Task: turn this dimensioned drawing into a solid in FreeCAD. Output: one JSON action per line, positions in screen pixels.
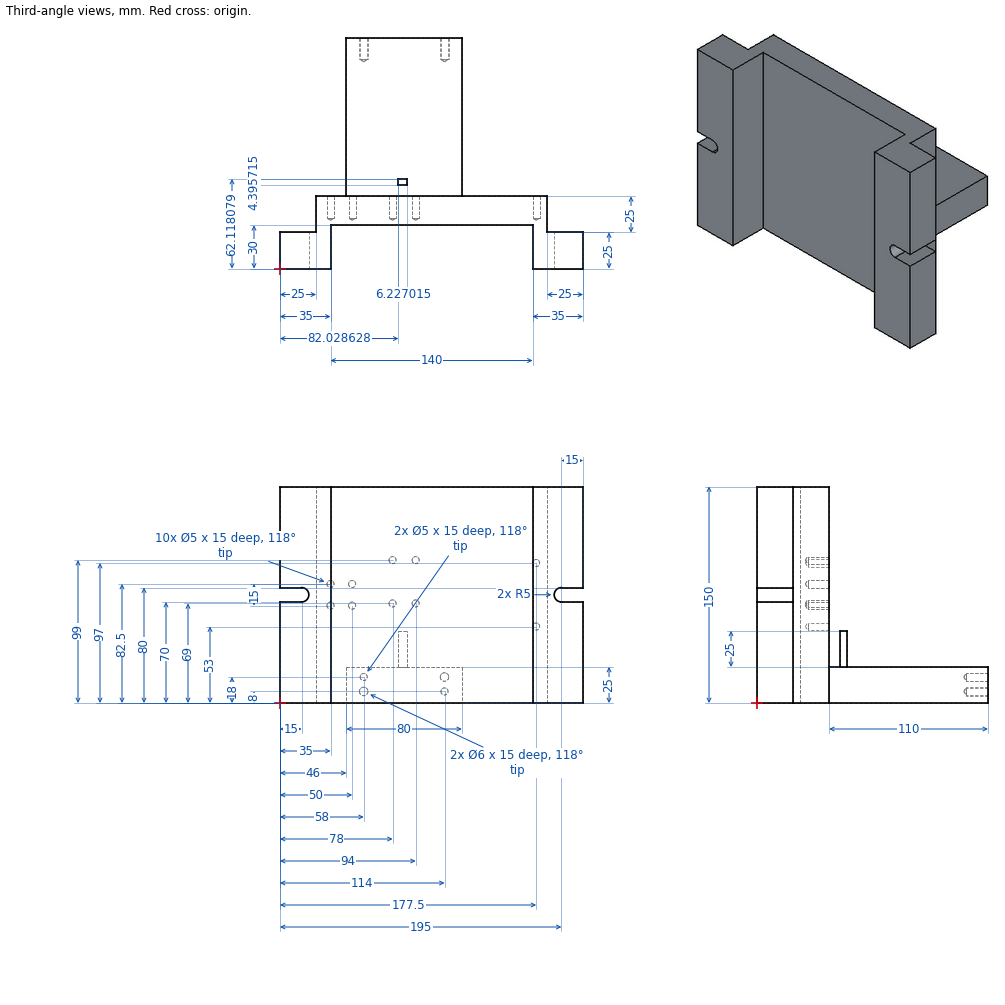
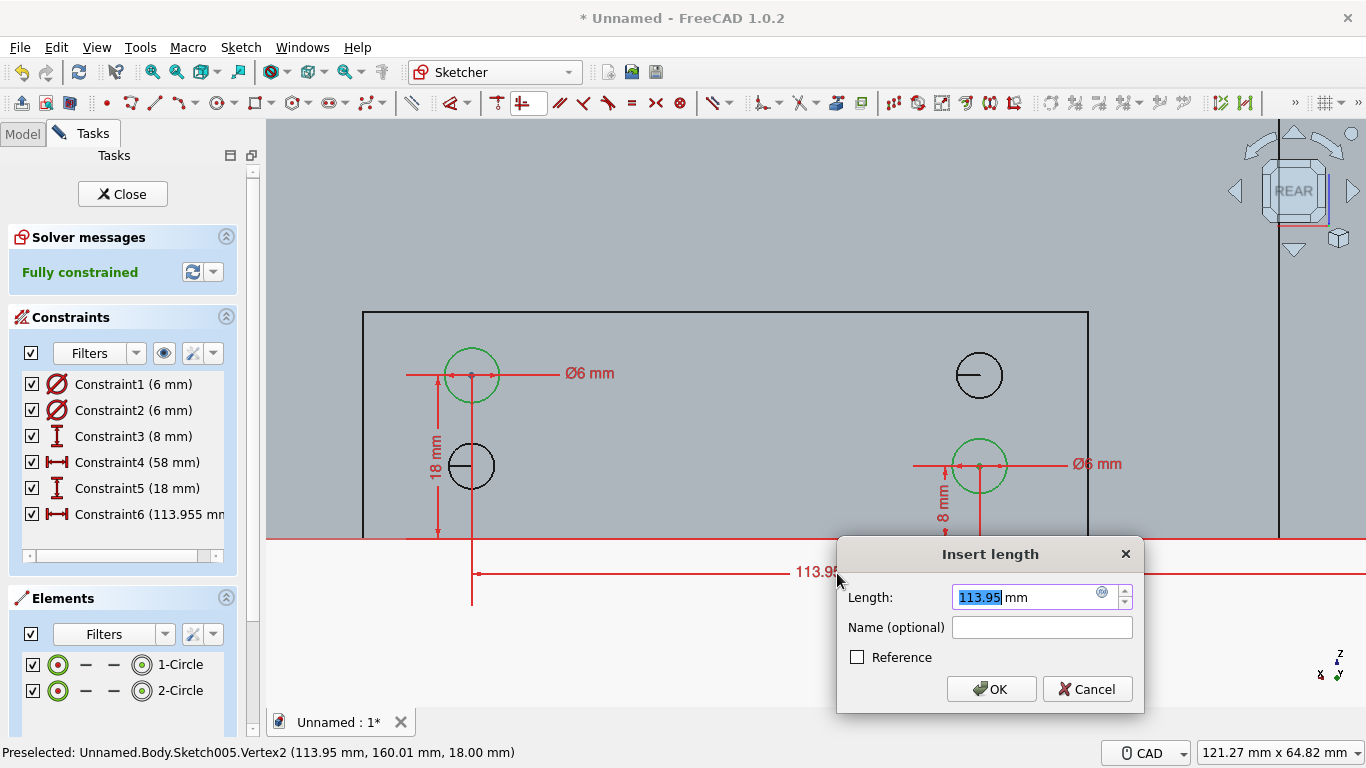
{"action": "type", "text": "114"}
{"action": "key", "text": "Return"}
{"action": "key", "text": "Escape"}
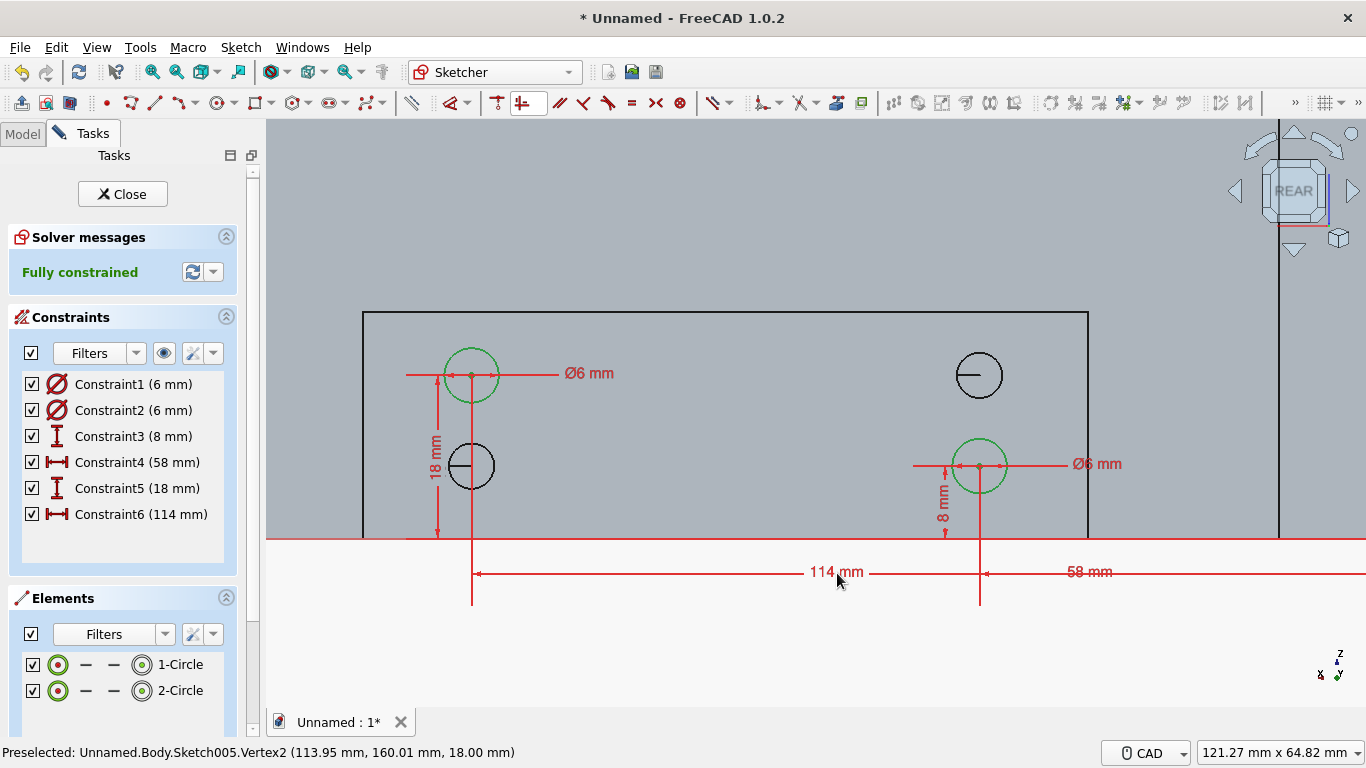
{"action": "left_click", "coordinate": [123, 194]}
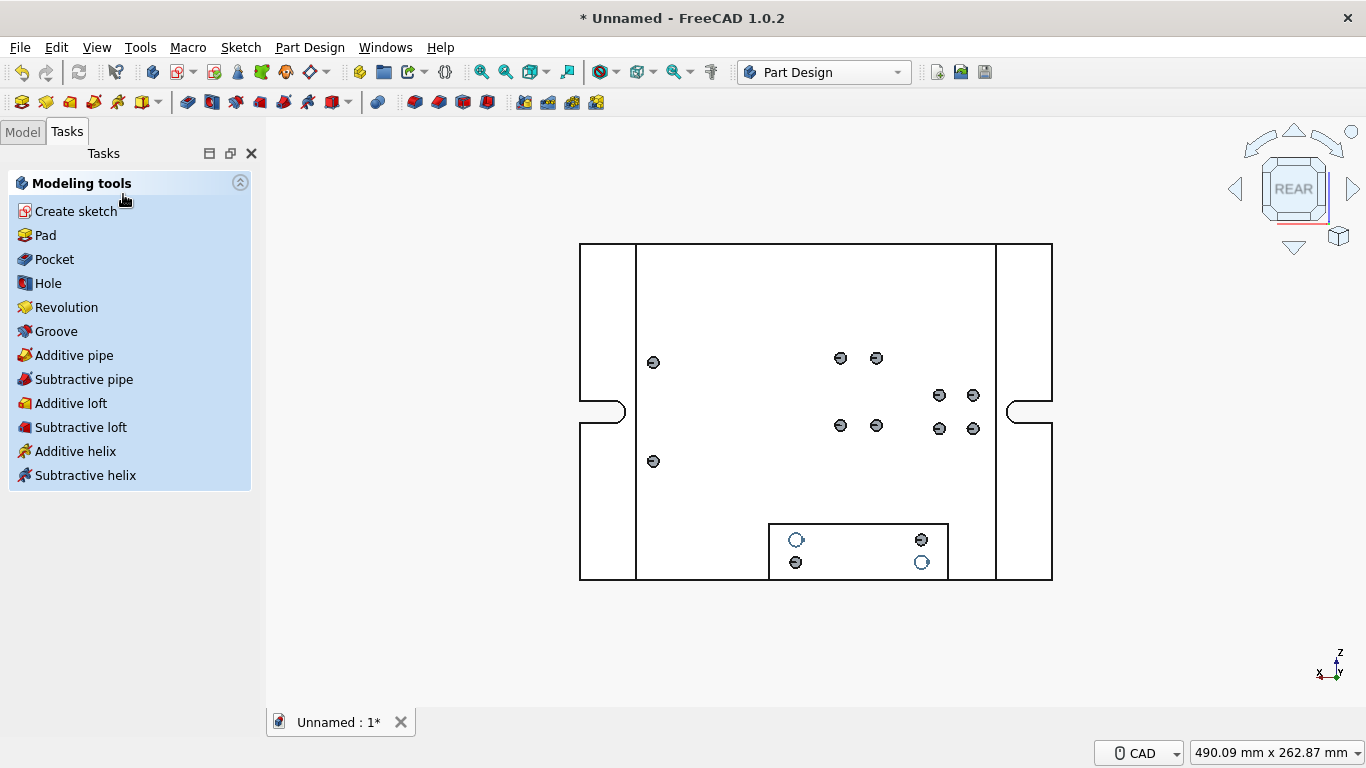
{"action": "left_click", "coordinate": [212, 102]}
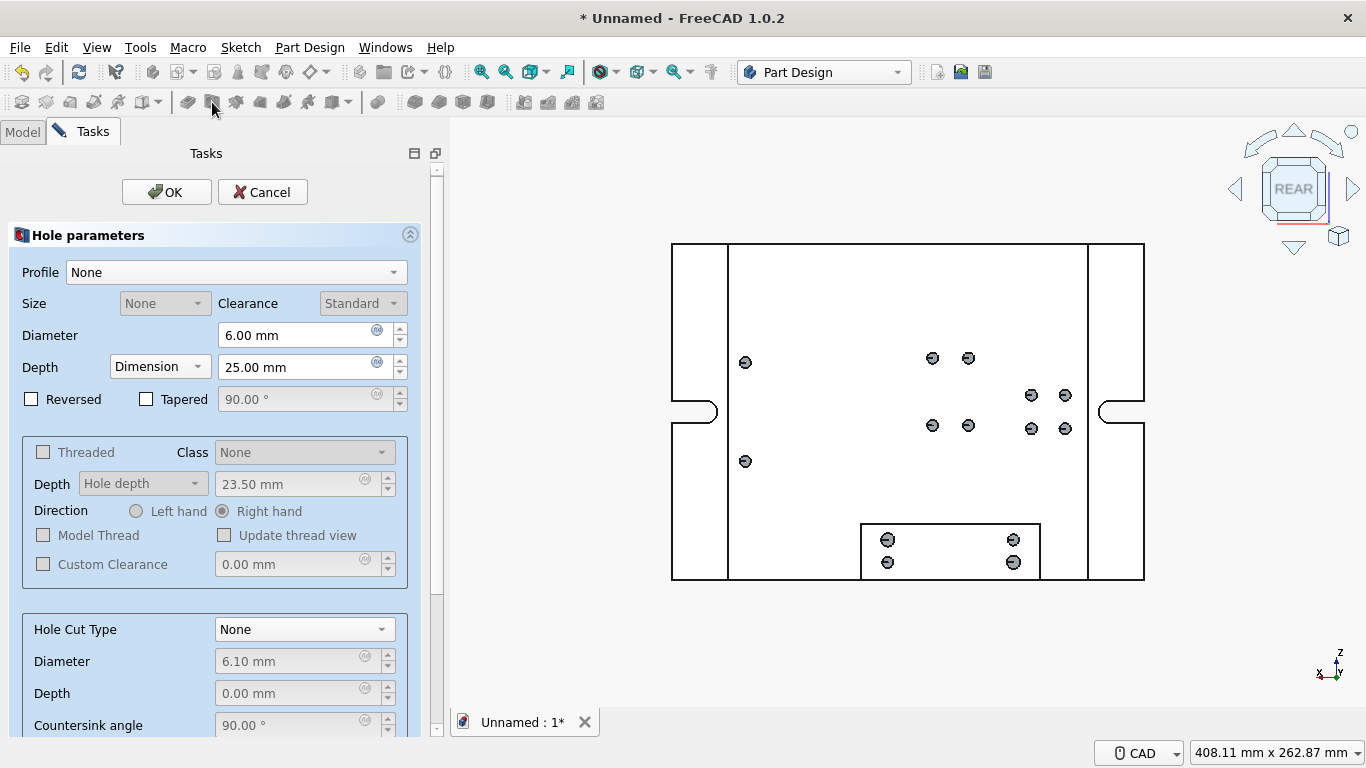
{"action": "triple_click", "coordinate": [305, 335]}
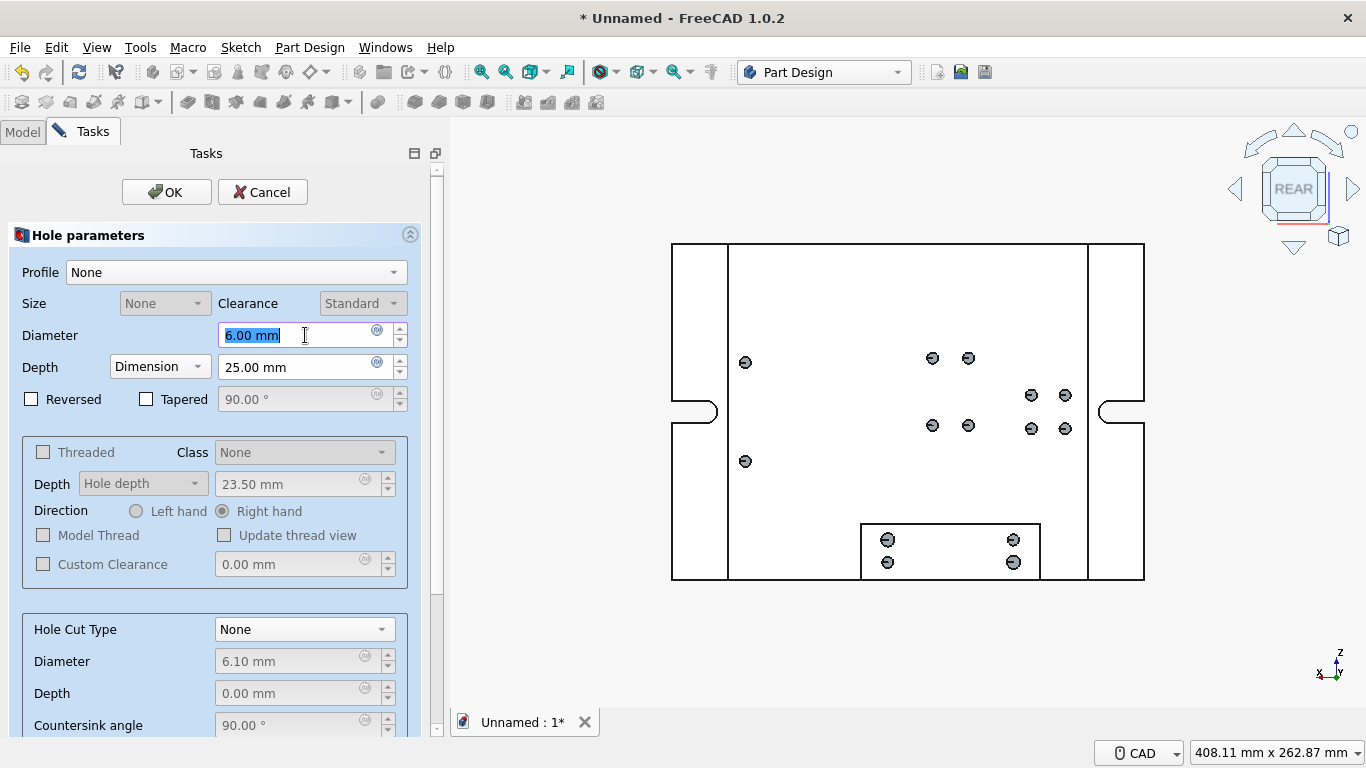
{"action": "type", "text": "6"}
{"action": "key", "text": "Tab"}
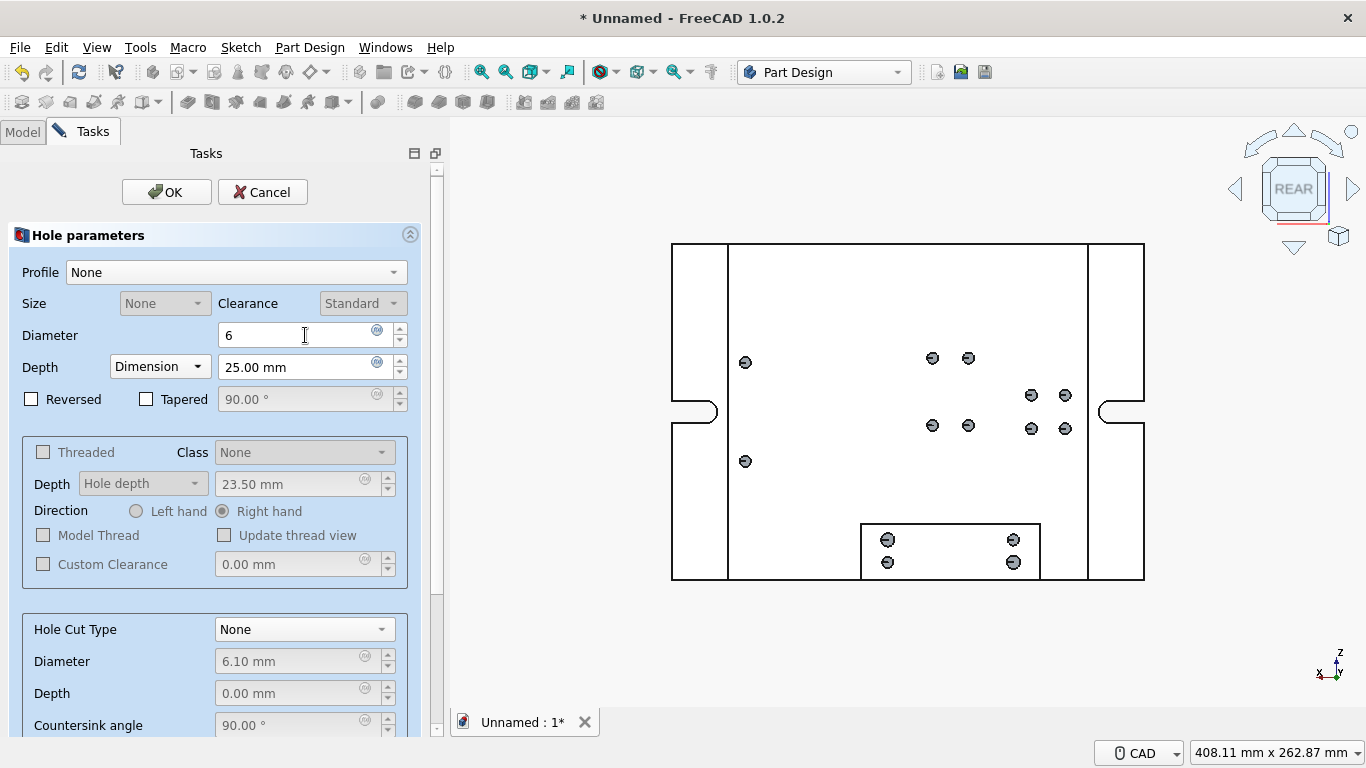
{"action": "triple_click", "coordinate": [305, 367]}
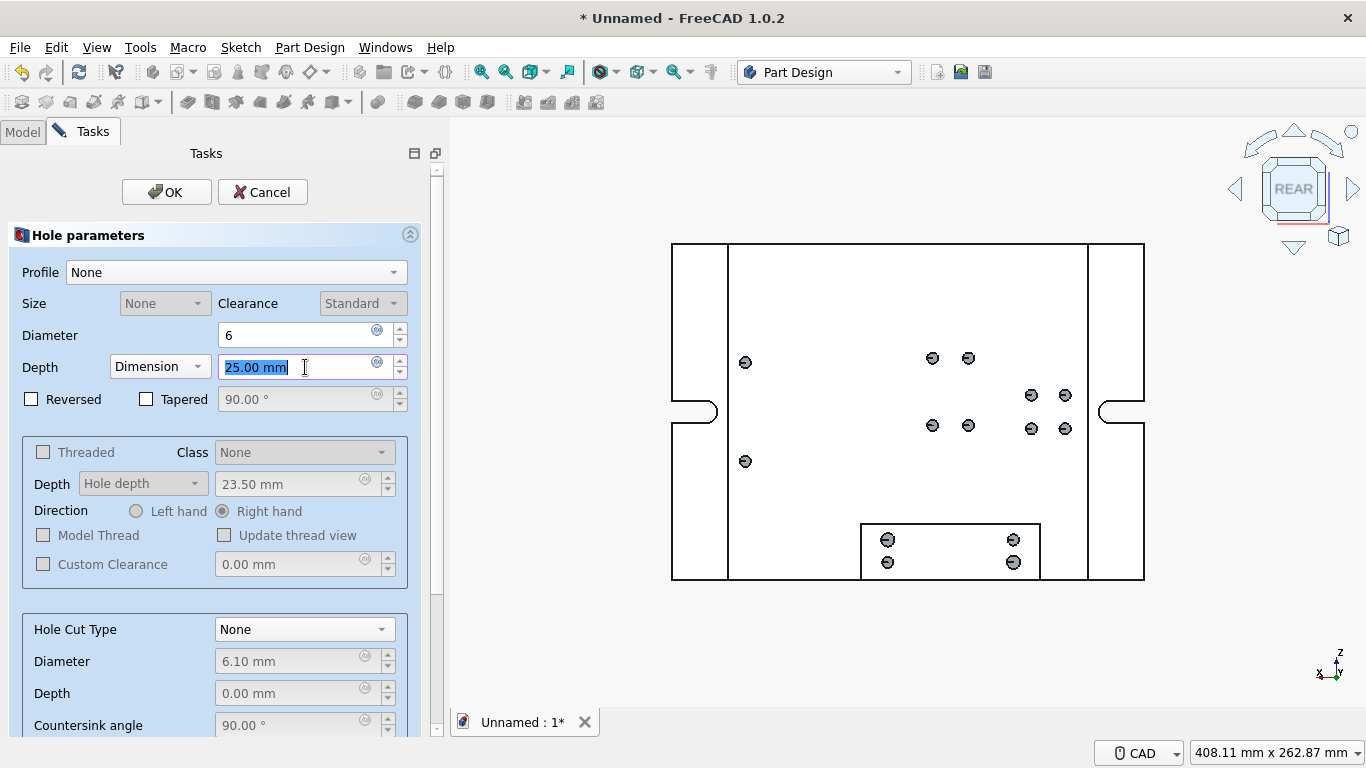
{"action": "type", "text": "15"}
{"action": "key", "text": "Tab"}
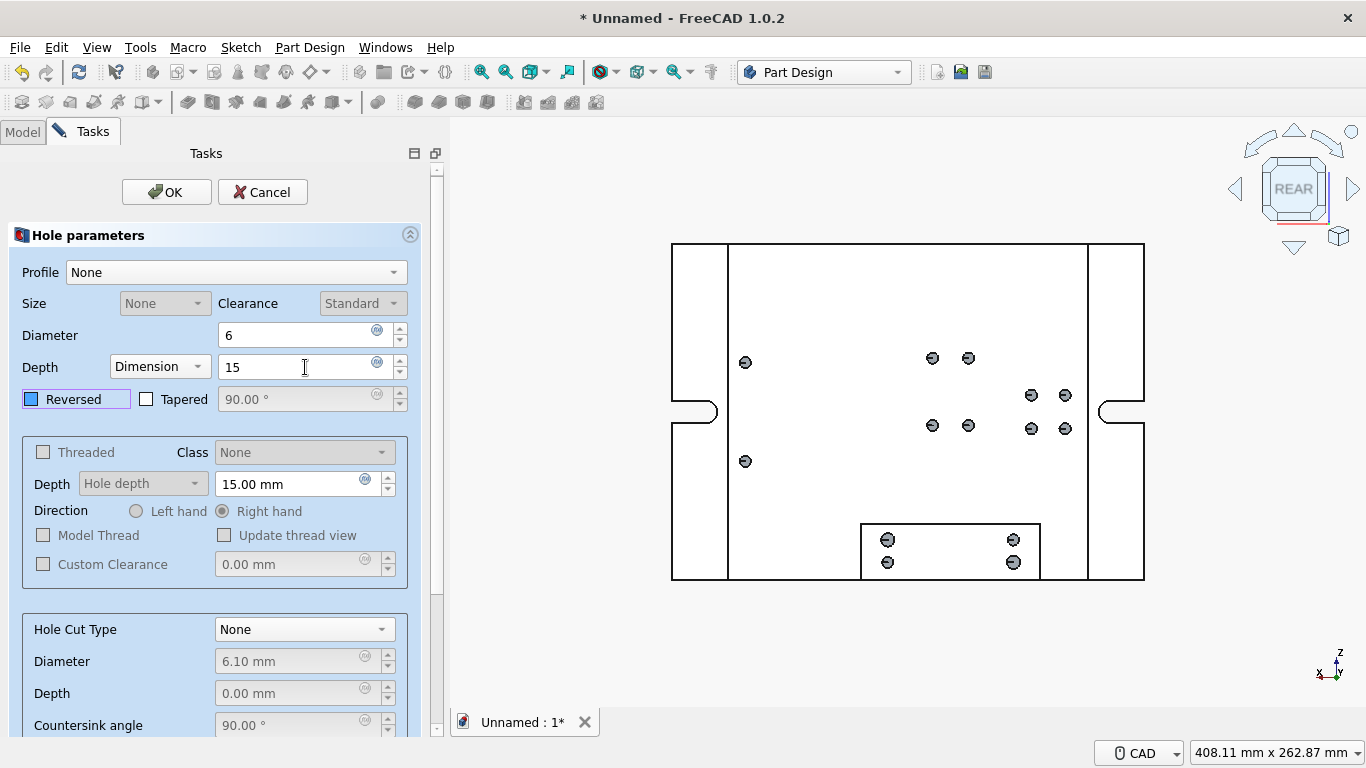
{"action": "left_click", "coordinate": [167, 192]}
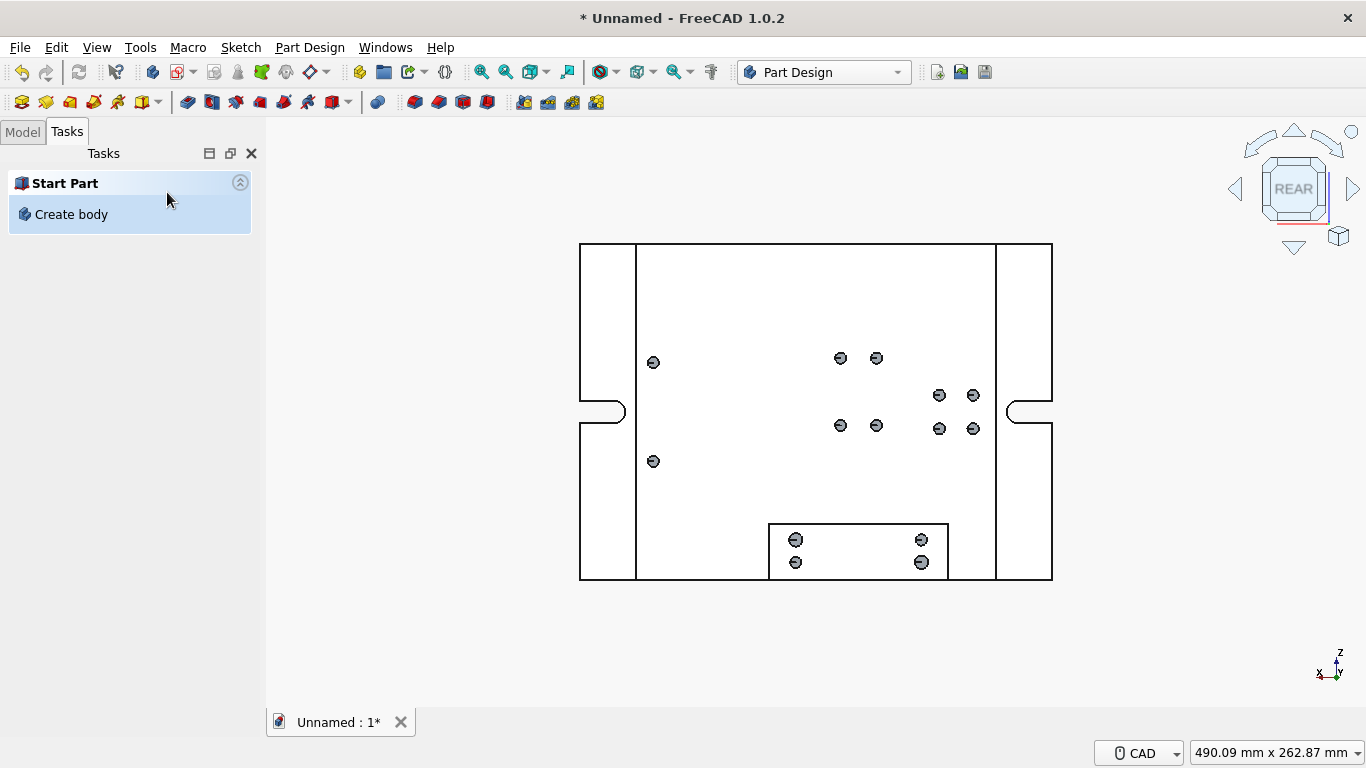
{"action": "key", "text": "0"}